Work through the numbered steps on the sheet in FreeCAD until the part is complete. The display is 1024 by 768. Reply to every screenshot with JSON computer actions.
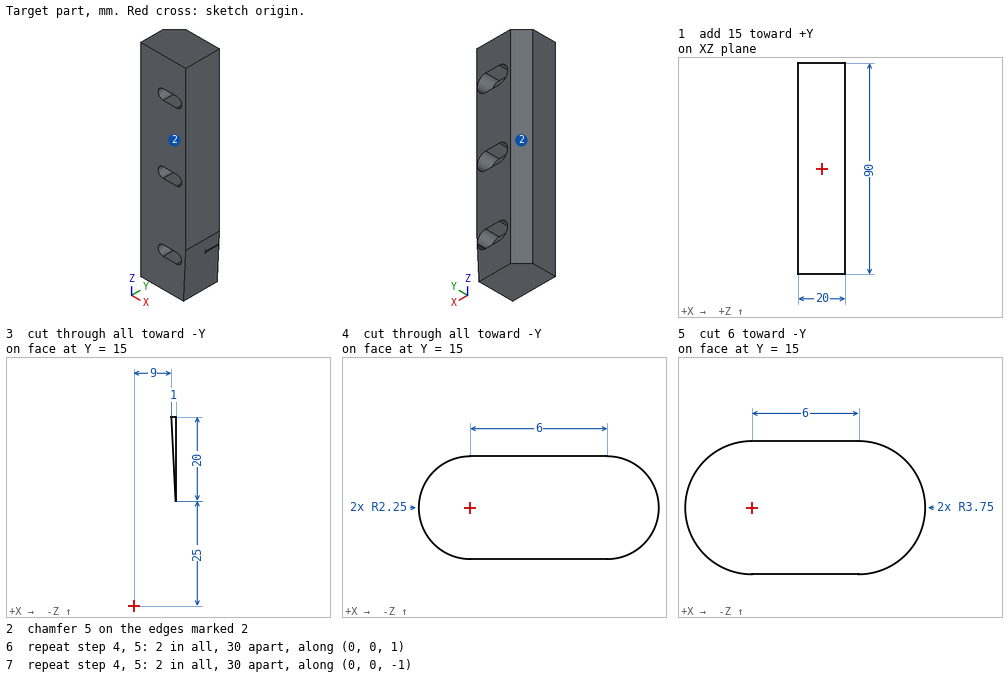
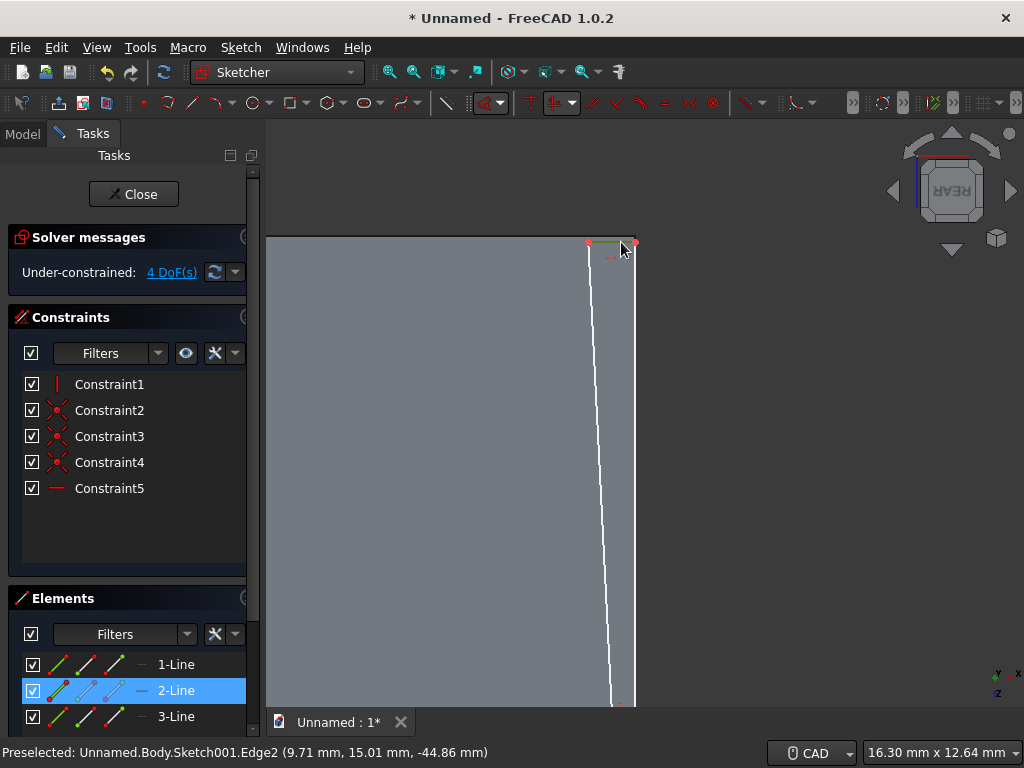
{"action": "left_click", "coordinate": [502, 104]}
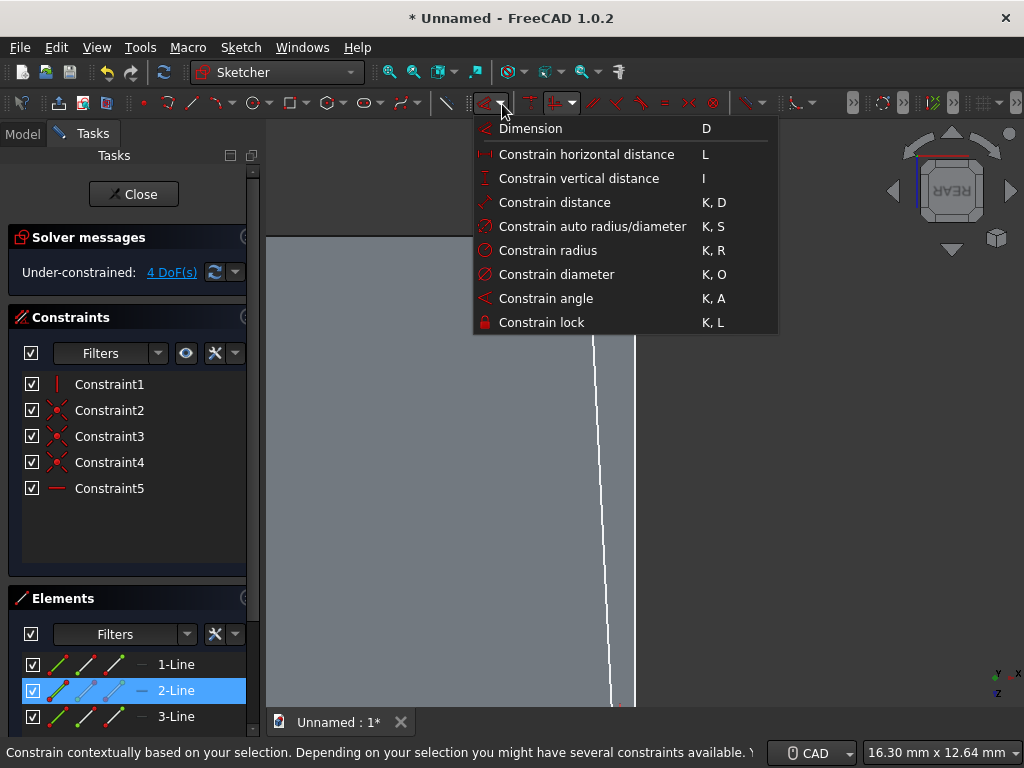
{"action": "left_click", "coordinate": [626, 154]}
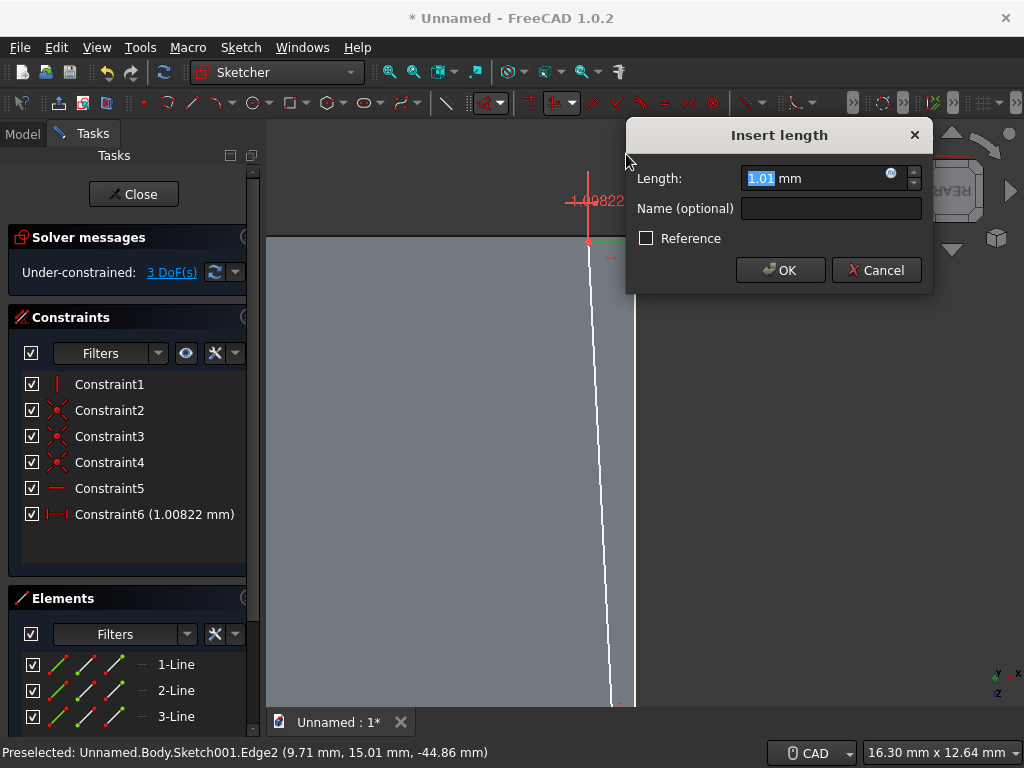
{"action": "type", "text": "1"}
{"action": "key", "text": "Return"}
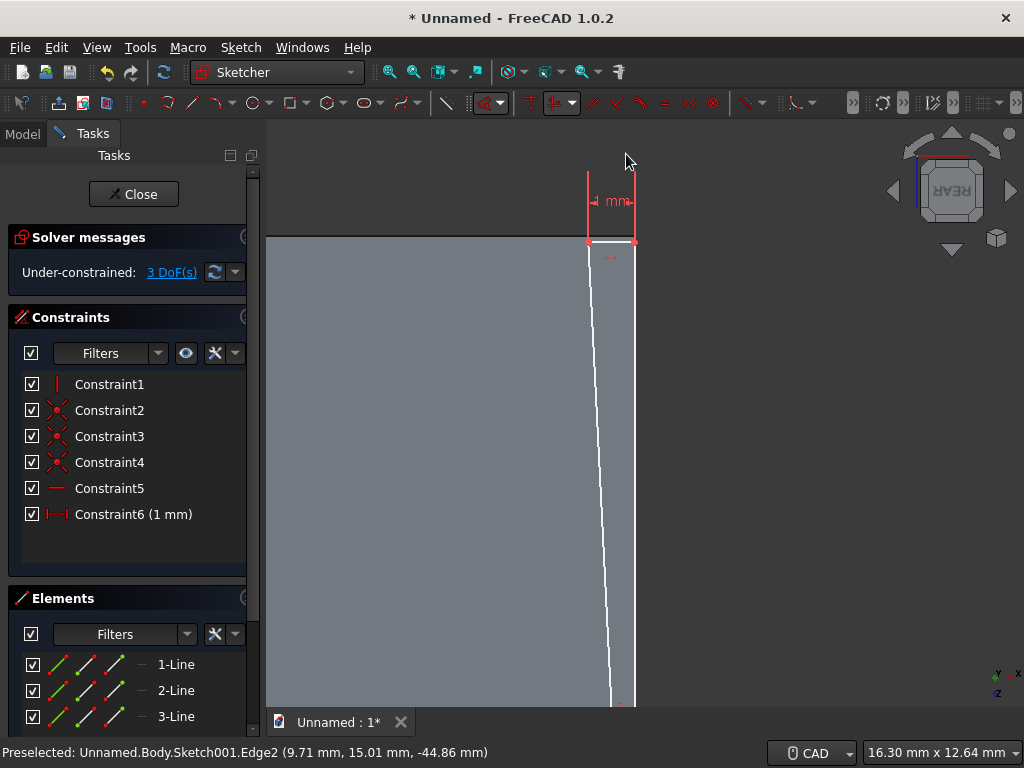
{"action": "left_click", "coordinate": [635, 522]}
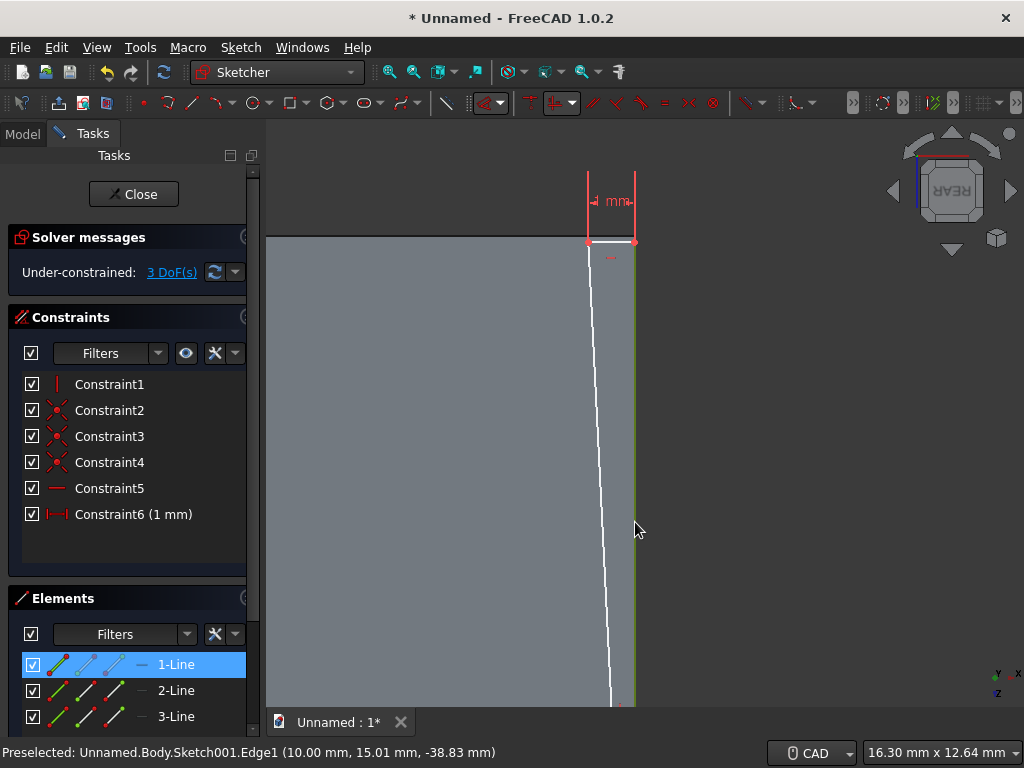
{"action": "key", "text": "i"}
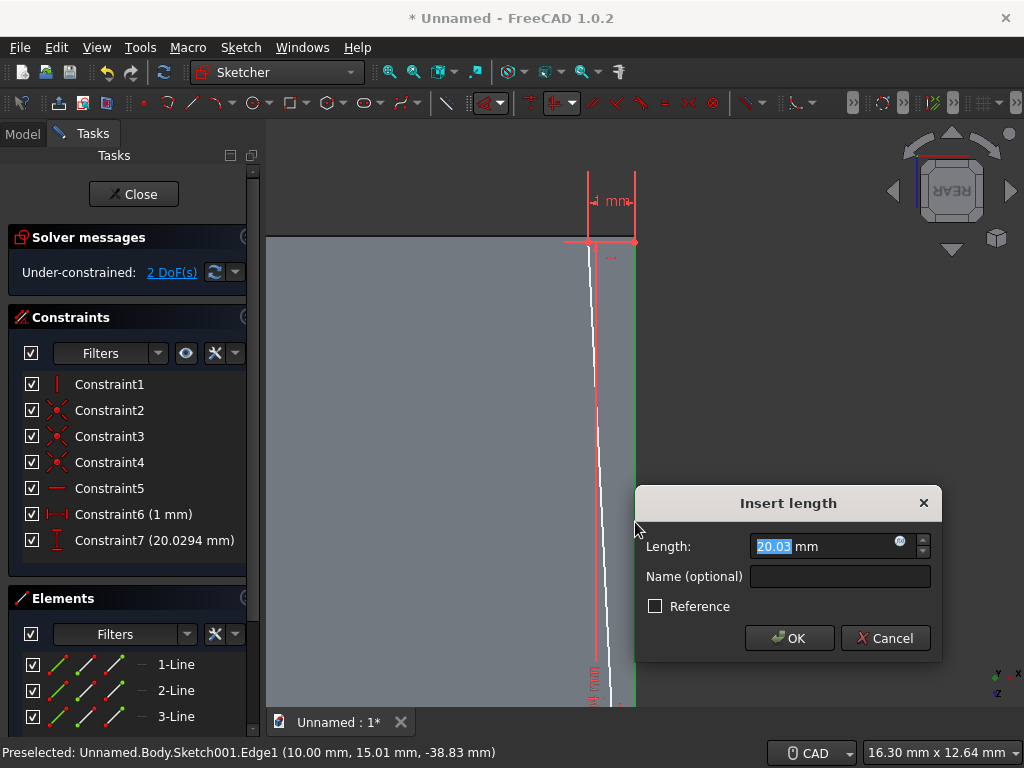
{"action": "type", "text": "20"}
{"action": "key", "text": "Return"}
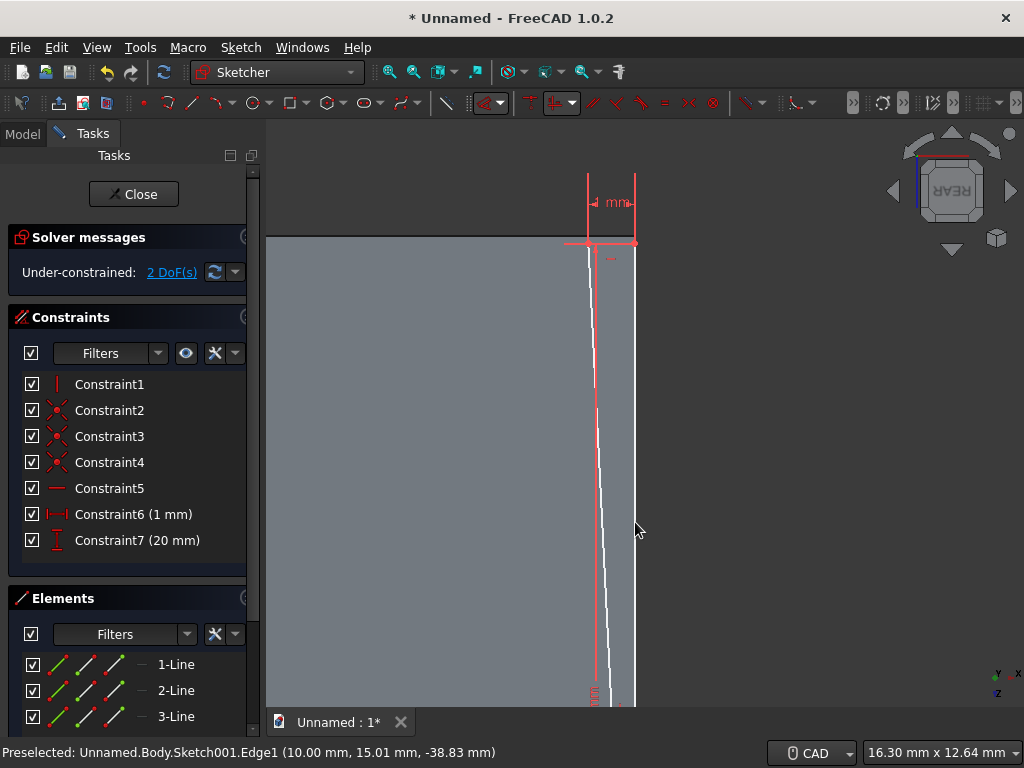
{"action": "scroll", "coordinate": [611, 241], "scroll_direction": "down", "scroll_amount": 9}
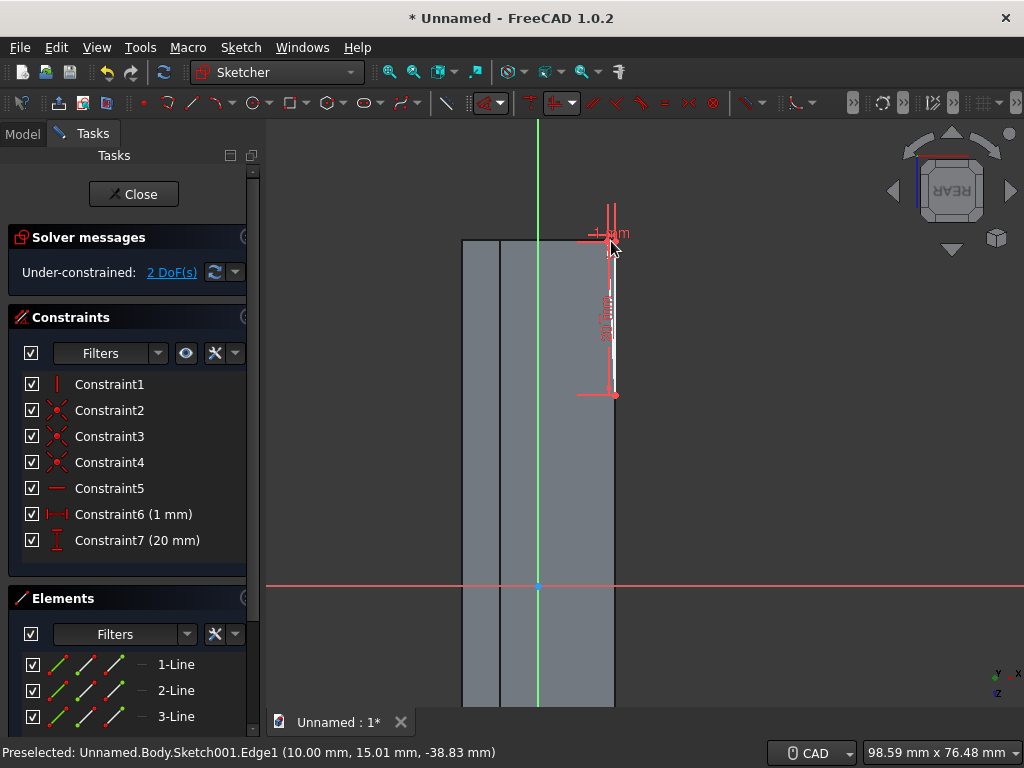
{"action": "scroll", "coordinate": [608, 242], "scroll_direction": "up", "scroll_amount": 3}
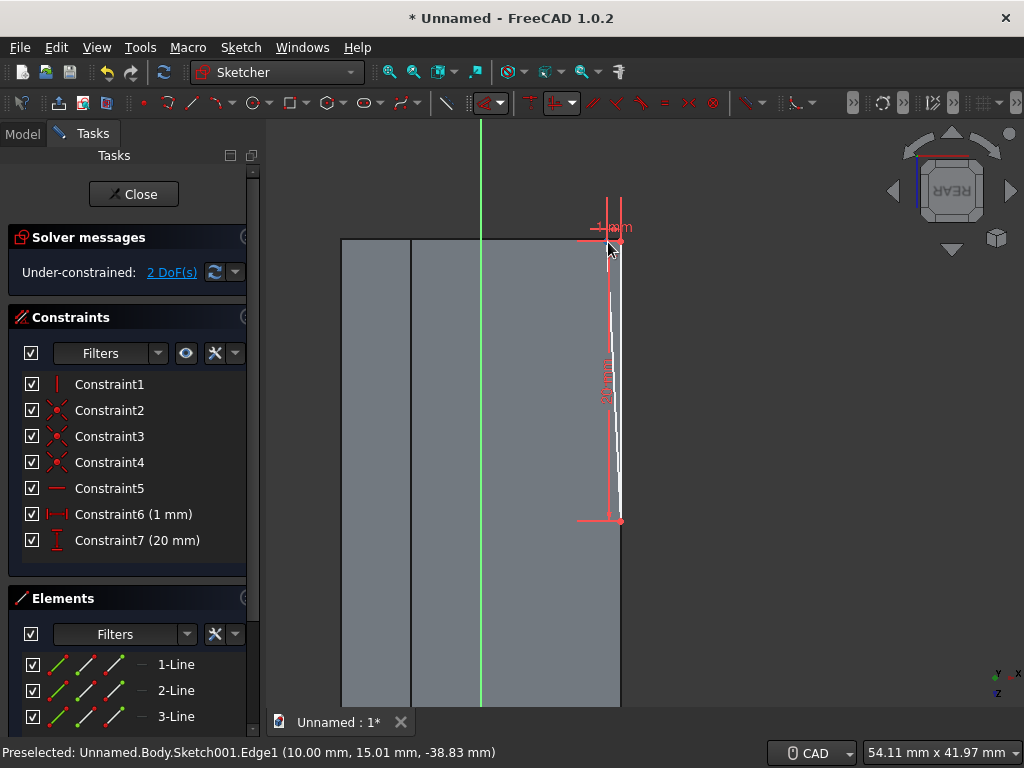
{"action": "left_click", "coordinate": [607, 241]}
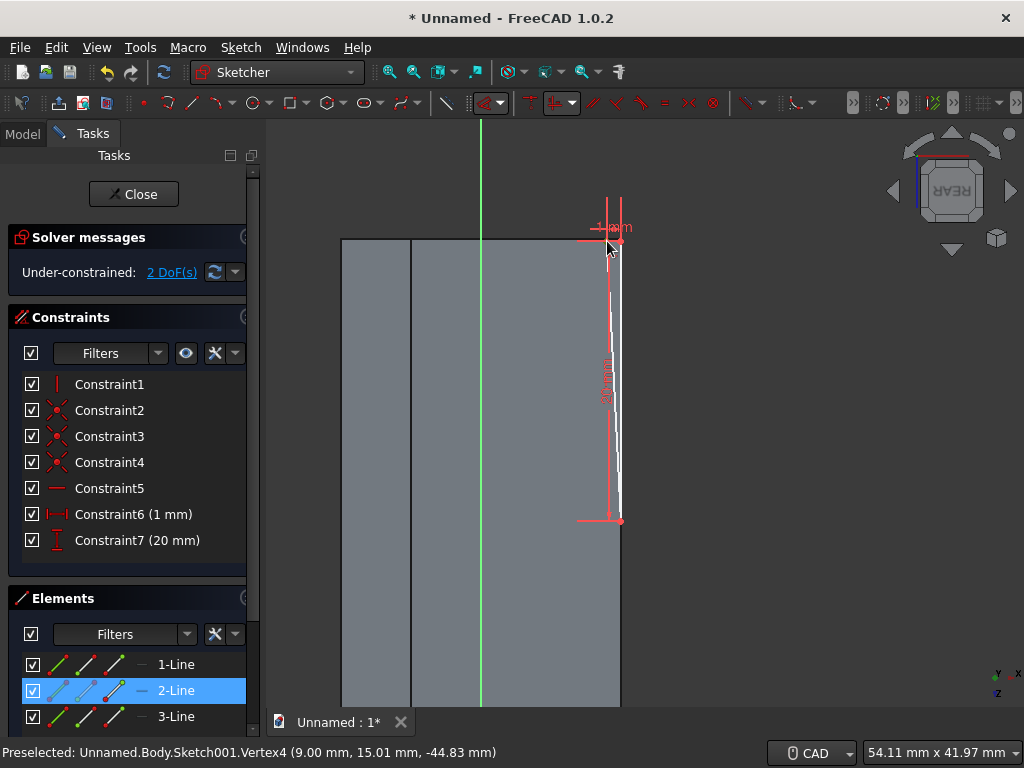
{"action": "left_click", "coordinate": [502, 104]}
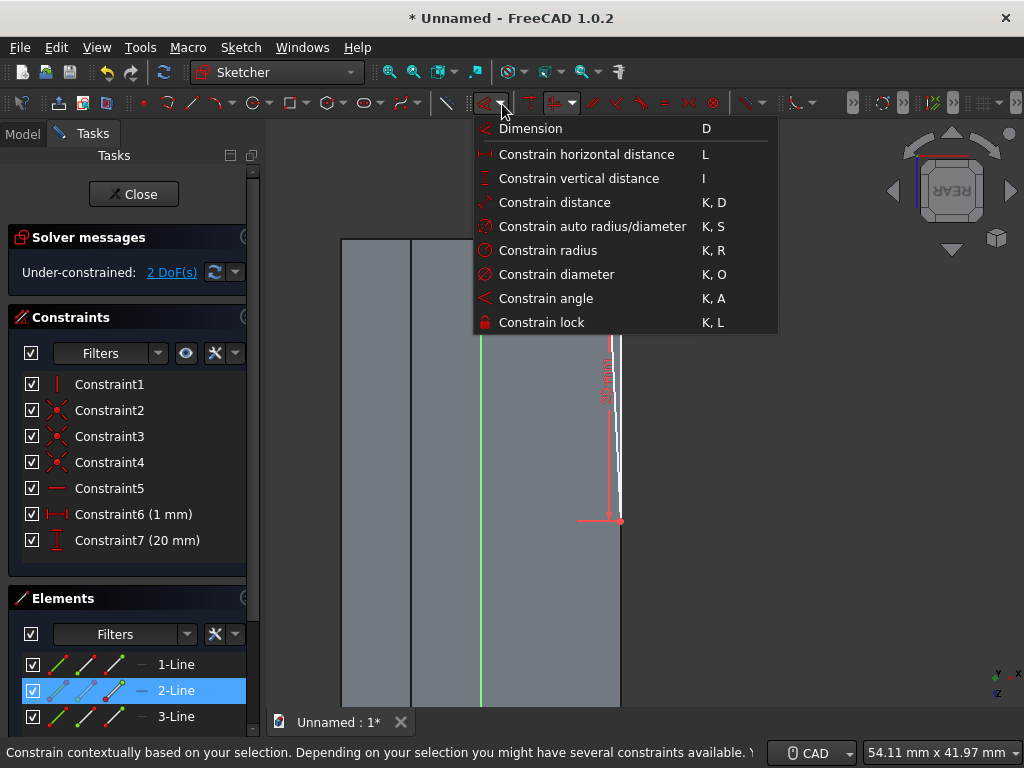
{"action": "left_click", "coordinate": [626, 154]}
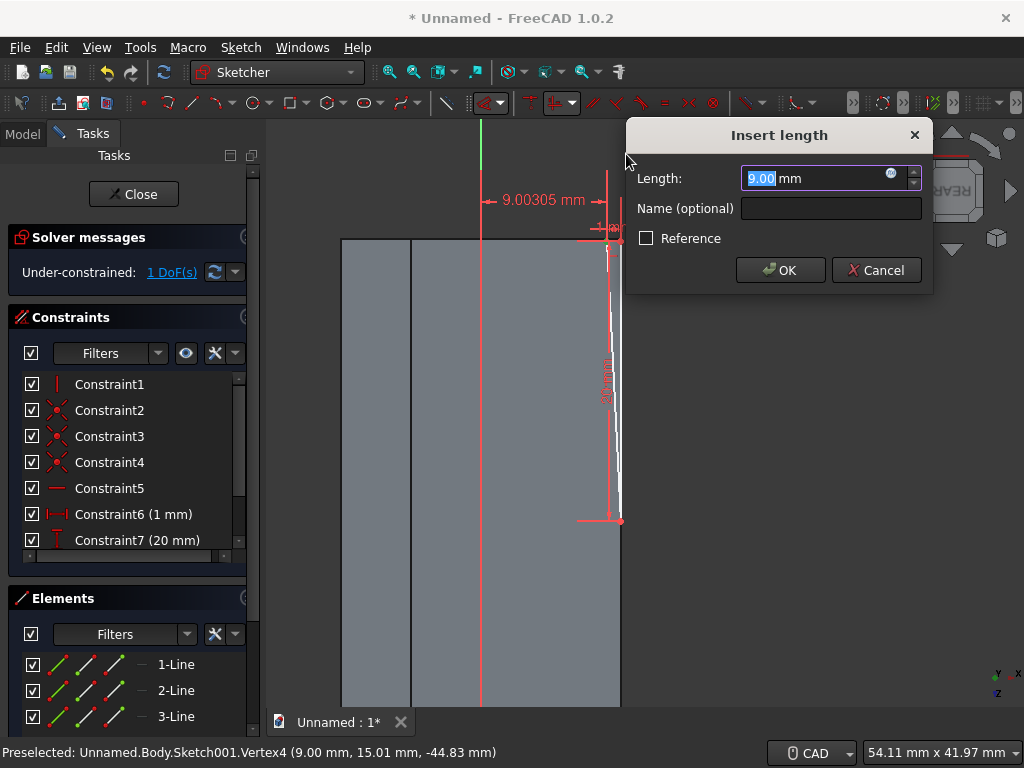
{"action": "type", "text": "9"}
{"action": "key", "text": "Return"}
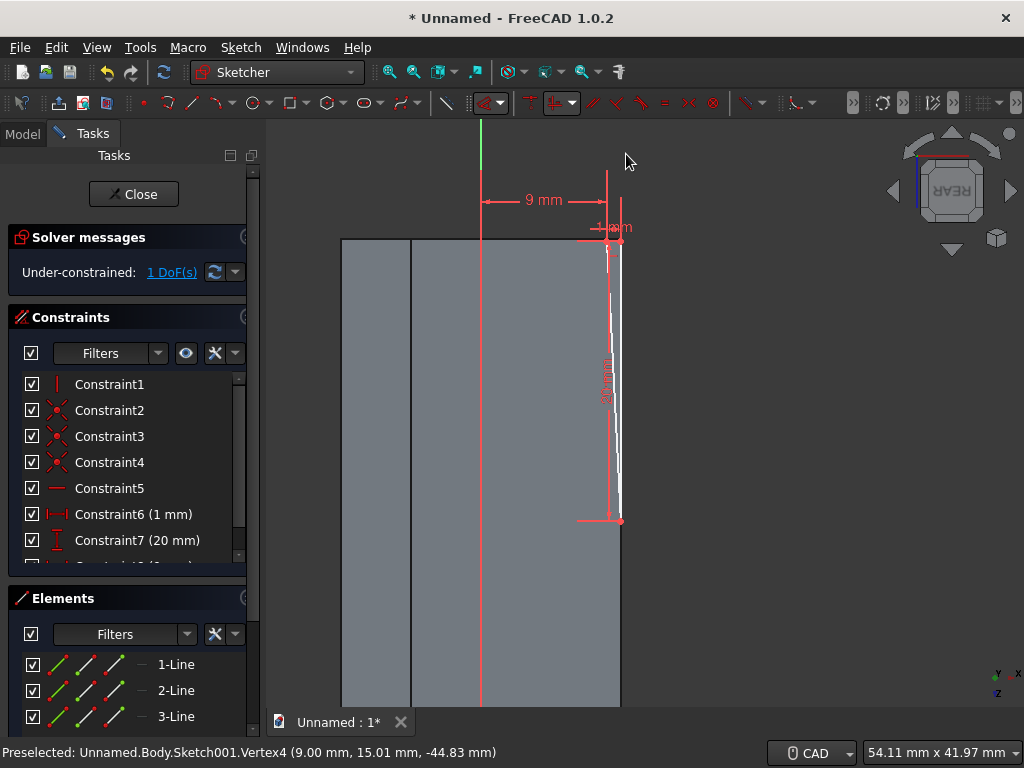
{"action": "left_click", "coordinate": [621, 521]}